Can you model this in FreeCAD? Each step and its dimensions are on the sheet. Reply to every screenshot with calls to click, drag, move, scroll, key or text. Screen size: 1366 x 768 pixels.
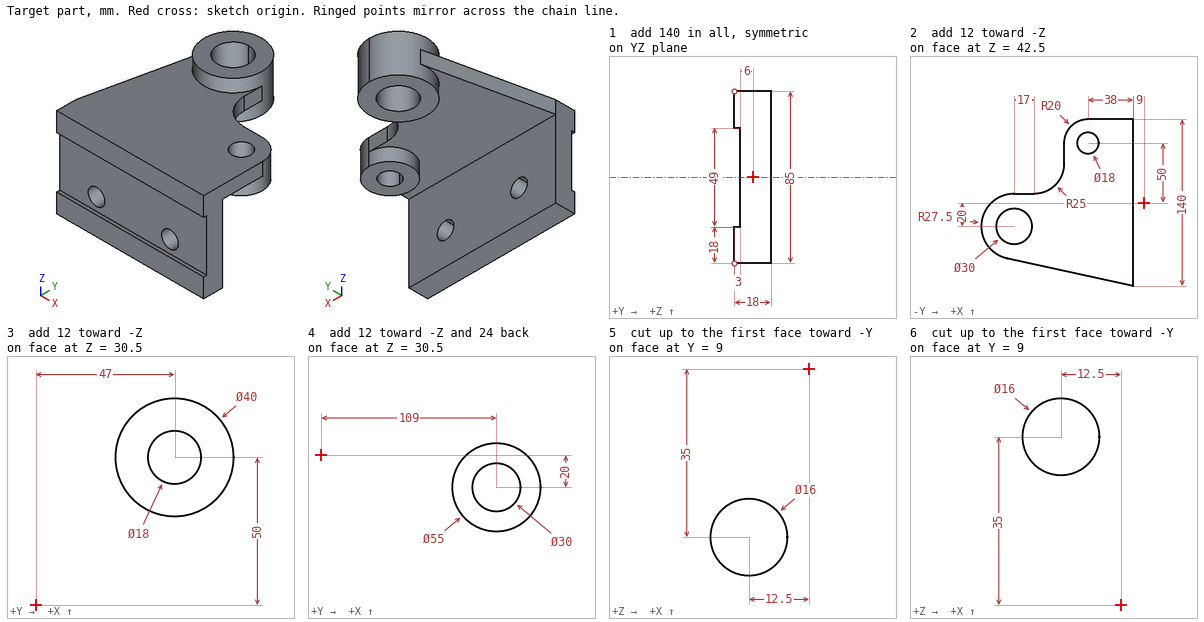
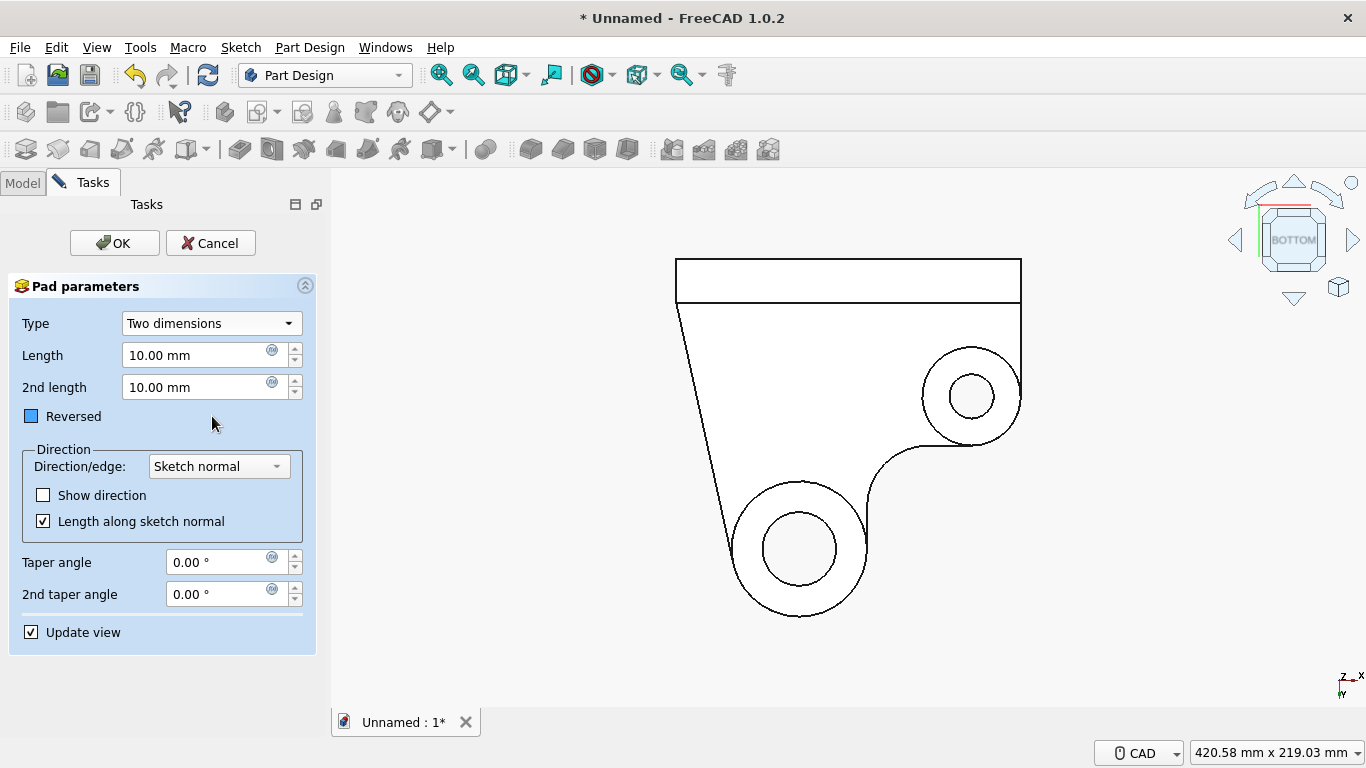
triple_click(204, 355)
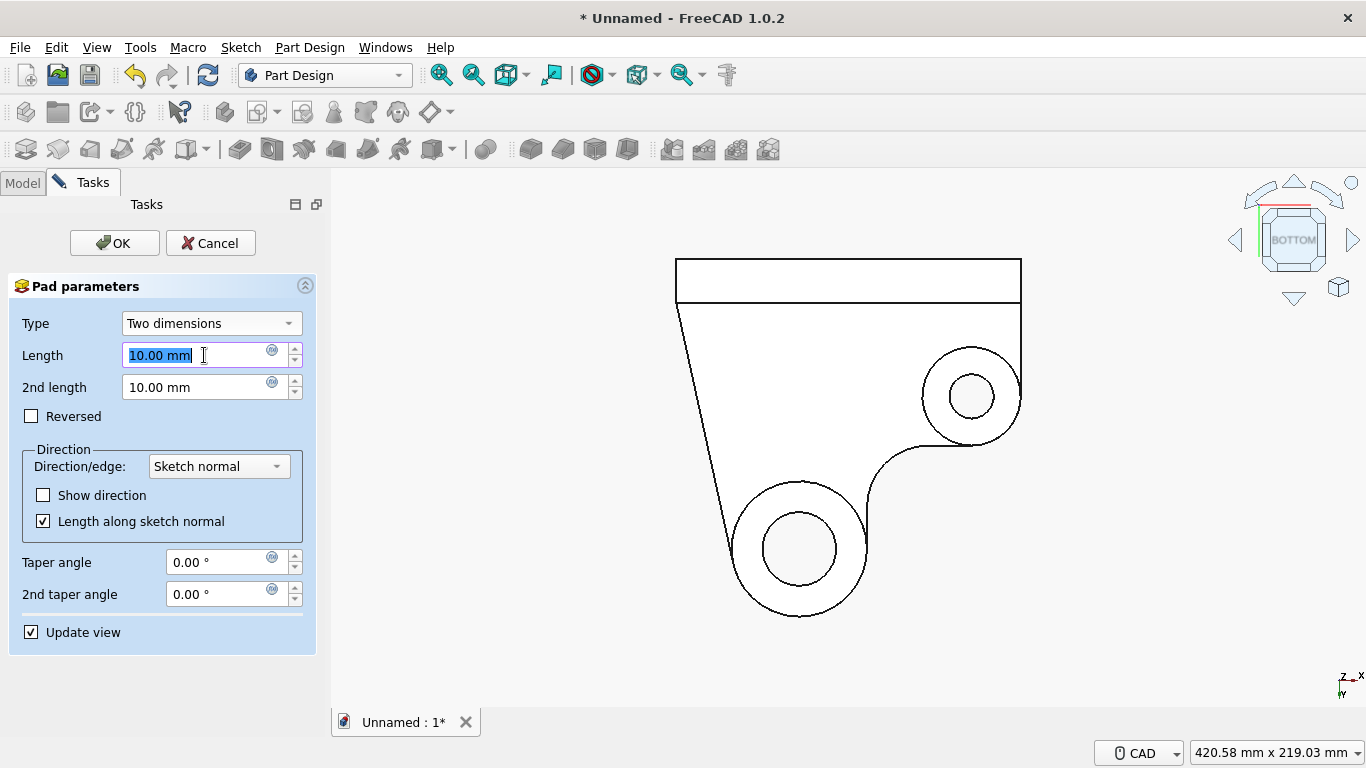
text(12)
key(Tab)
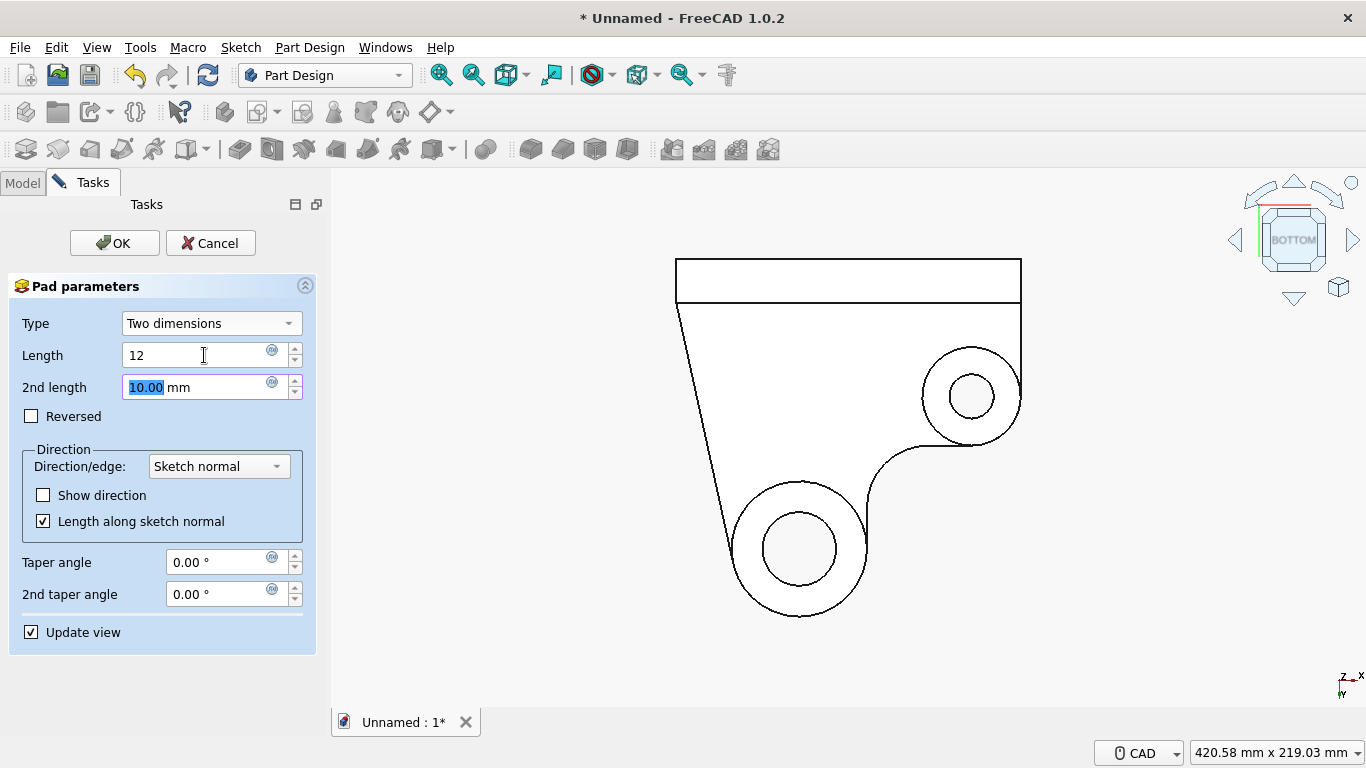
text(24)
key(Tab)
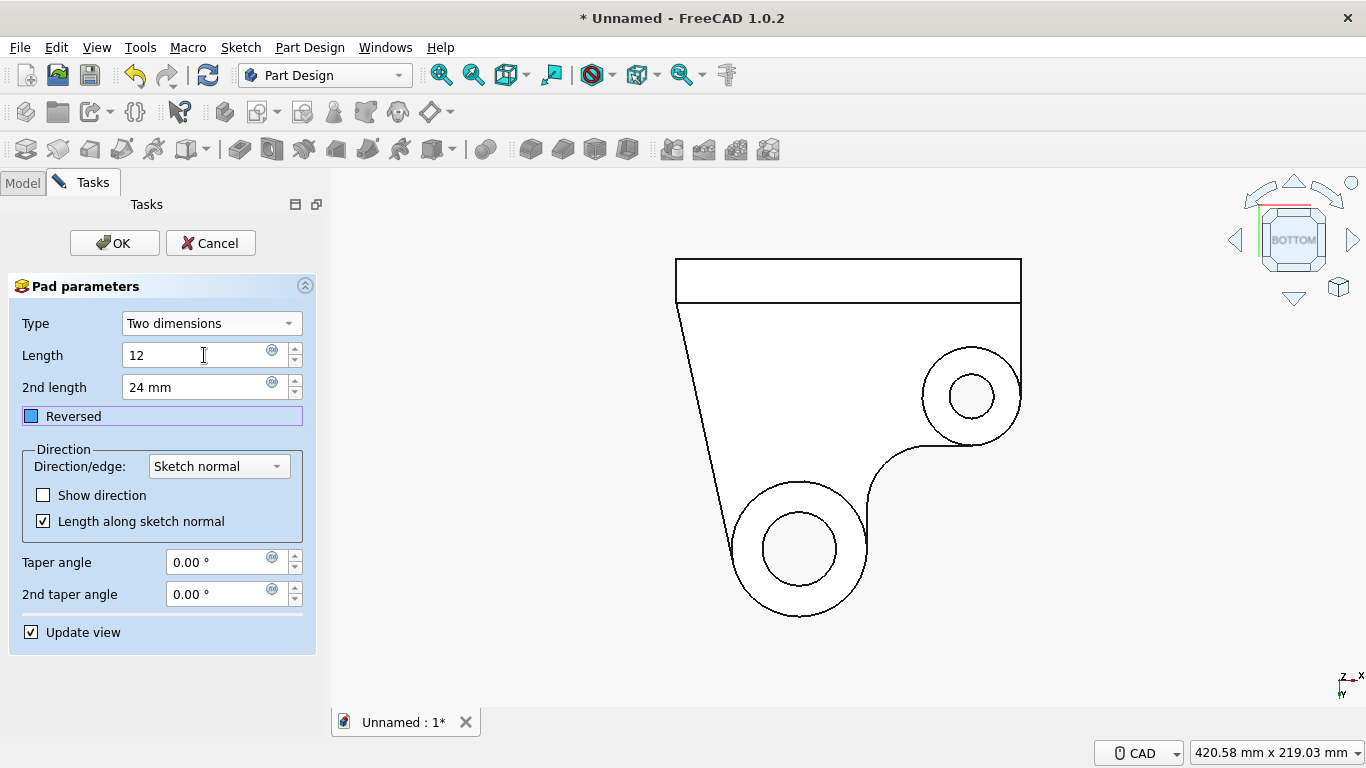
click(115, 243)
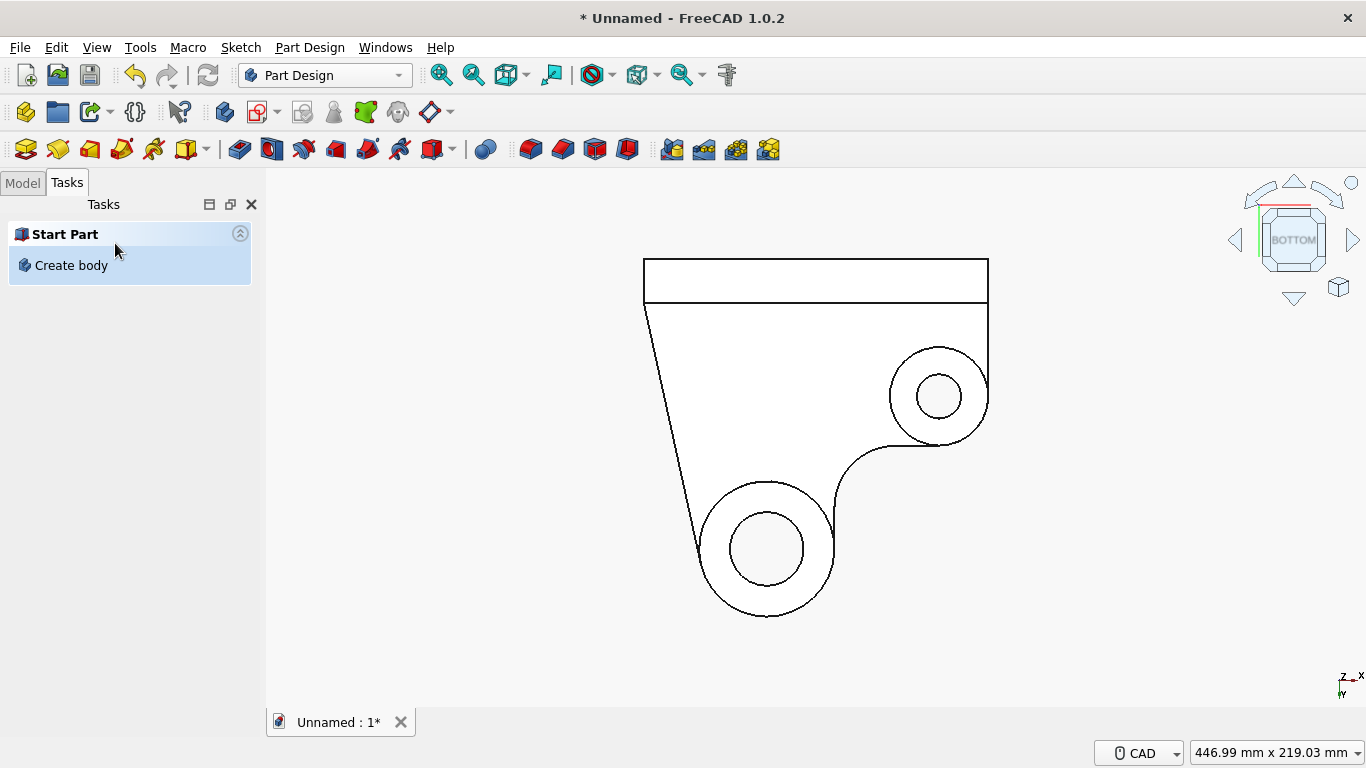
key(4)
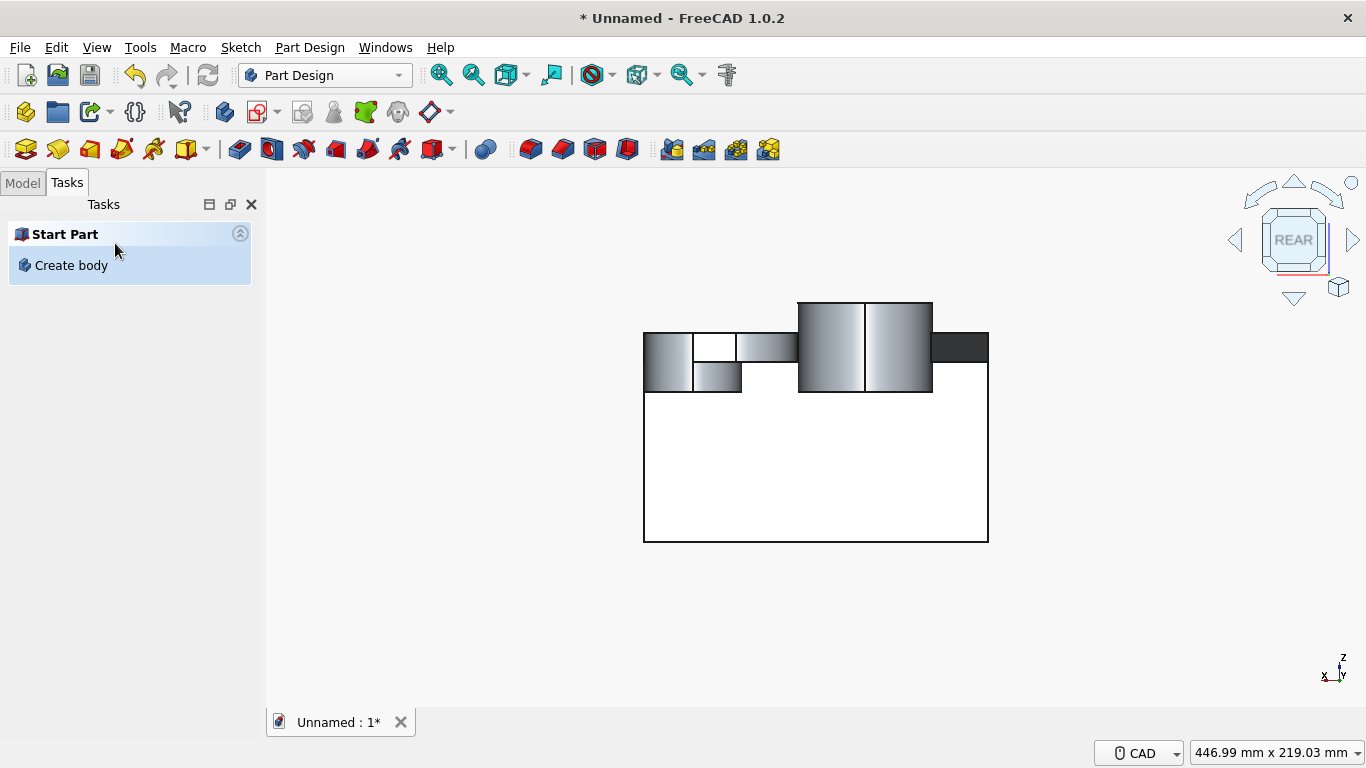
key(v)
key(f)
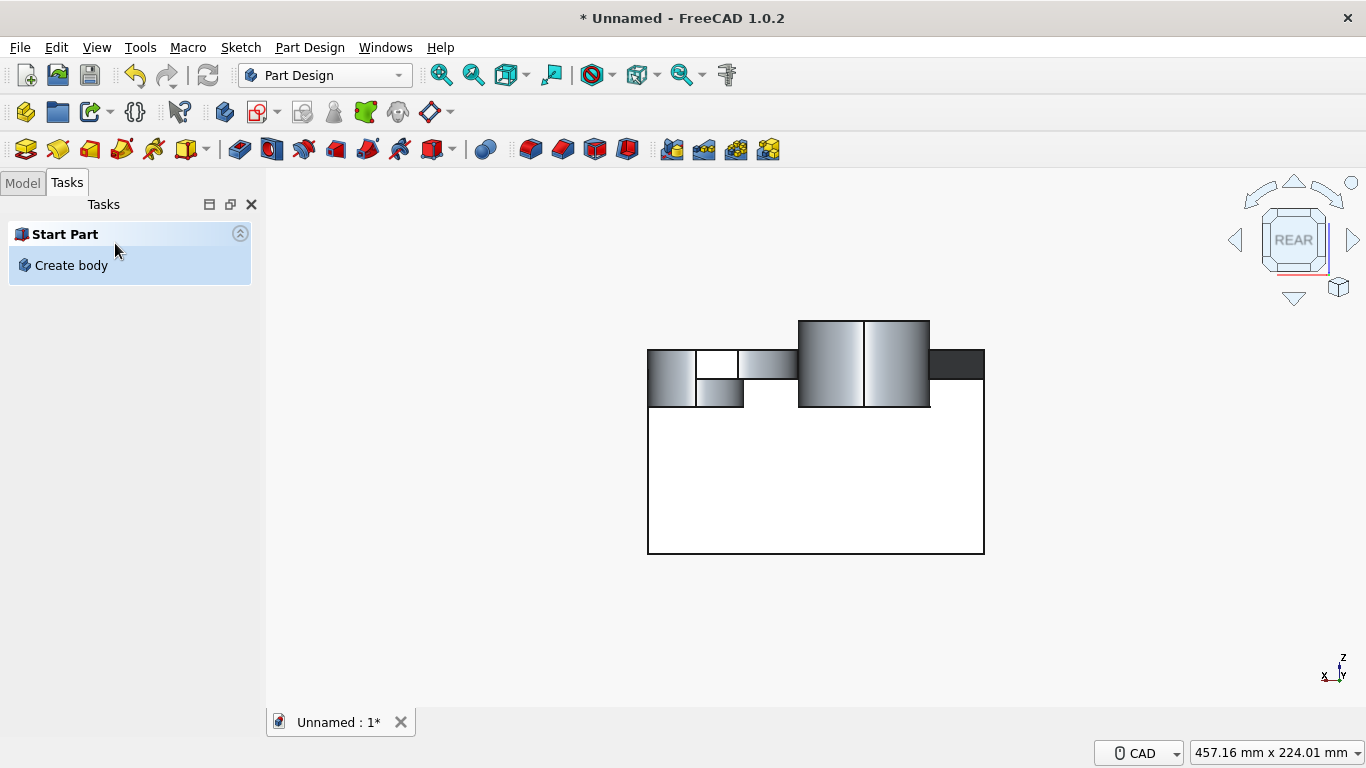
click(864, 465)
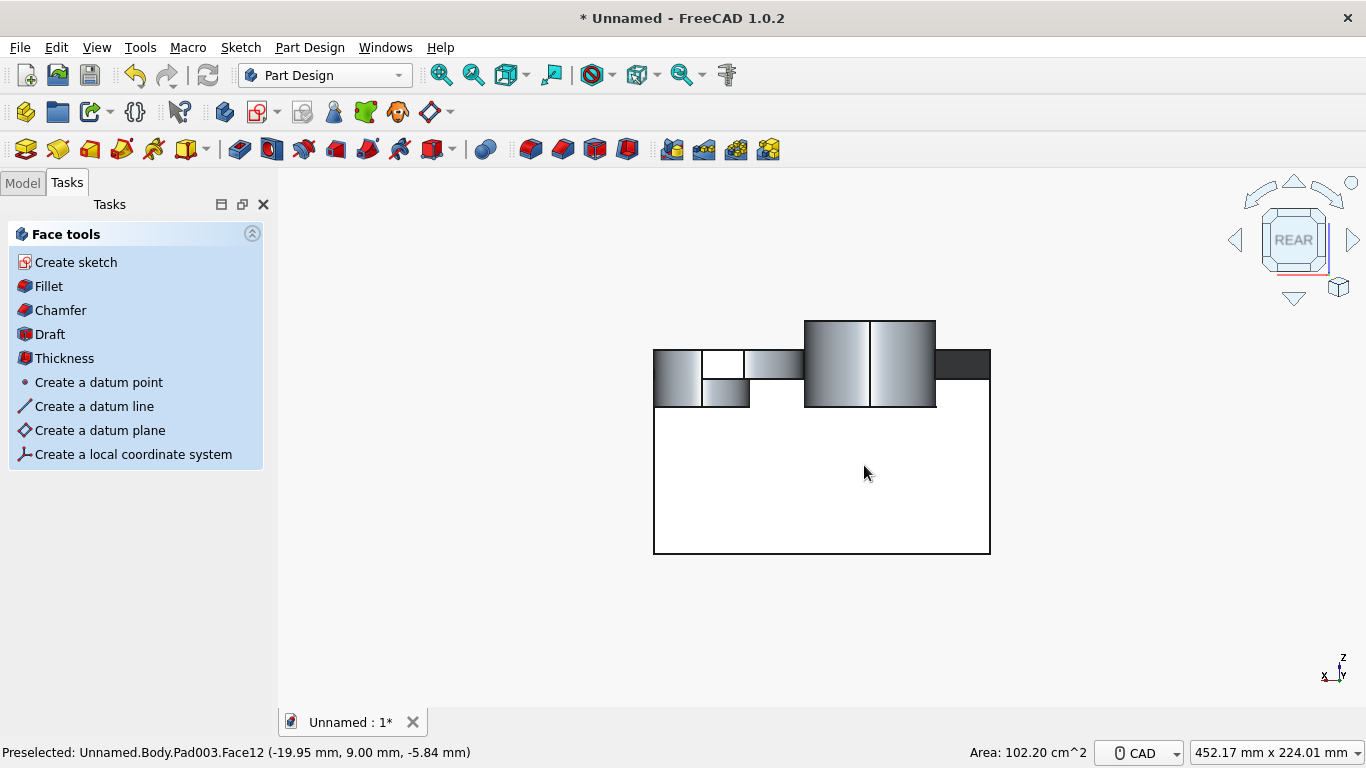
click(258, 112)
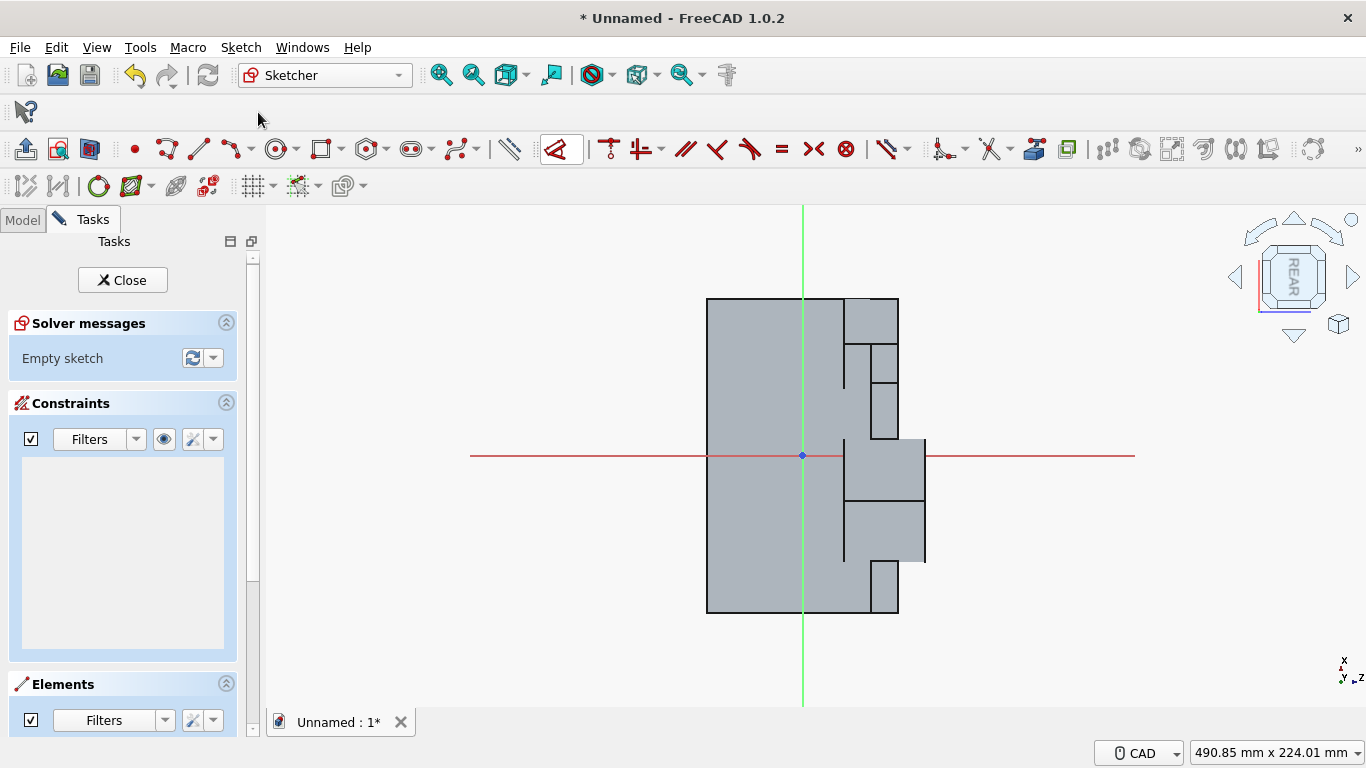
click(90, 150)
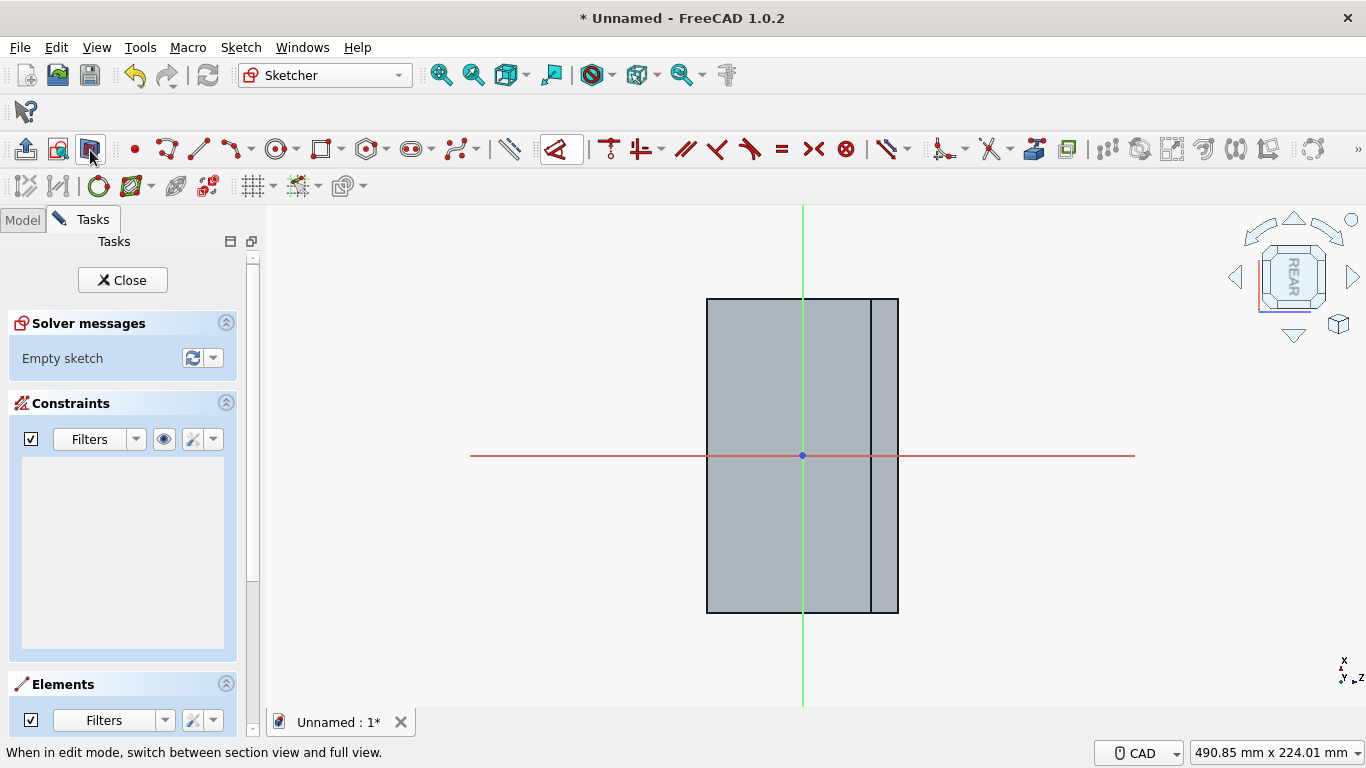
scroll(778, 544, up, 11)